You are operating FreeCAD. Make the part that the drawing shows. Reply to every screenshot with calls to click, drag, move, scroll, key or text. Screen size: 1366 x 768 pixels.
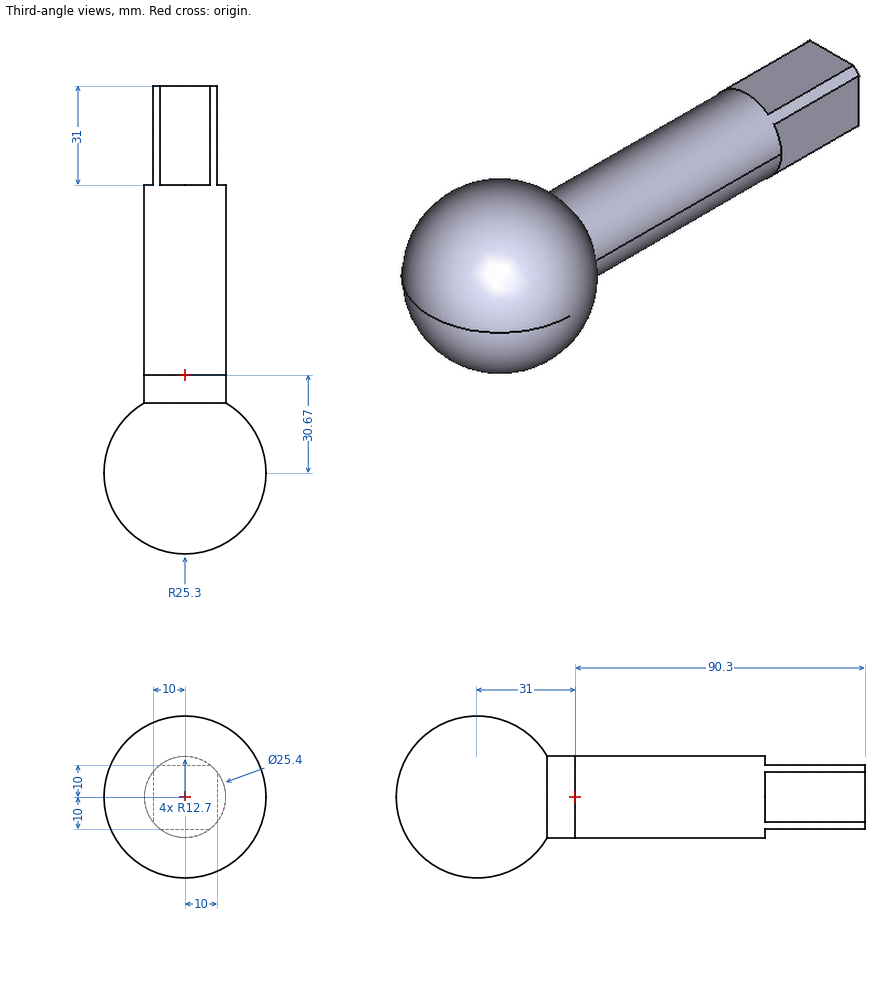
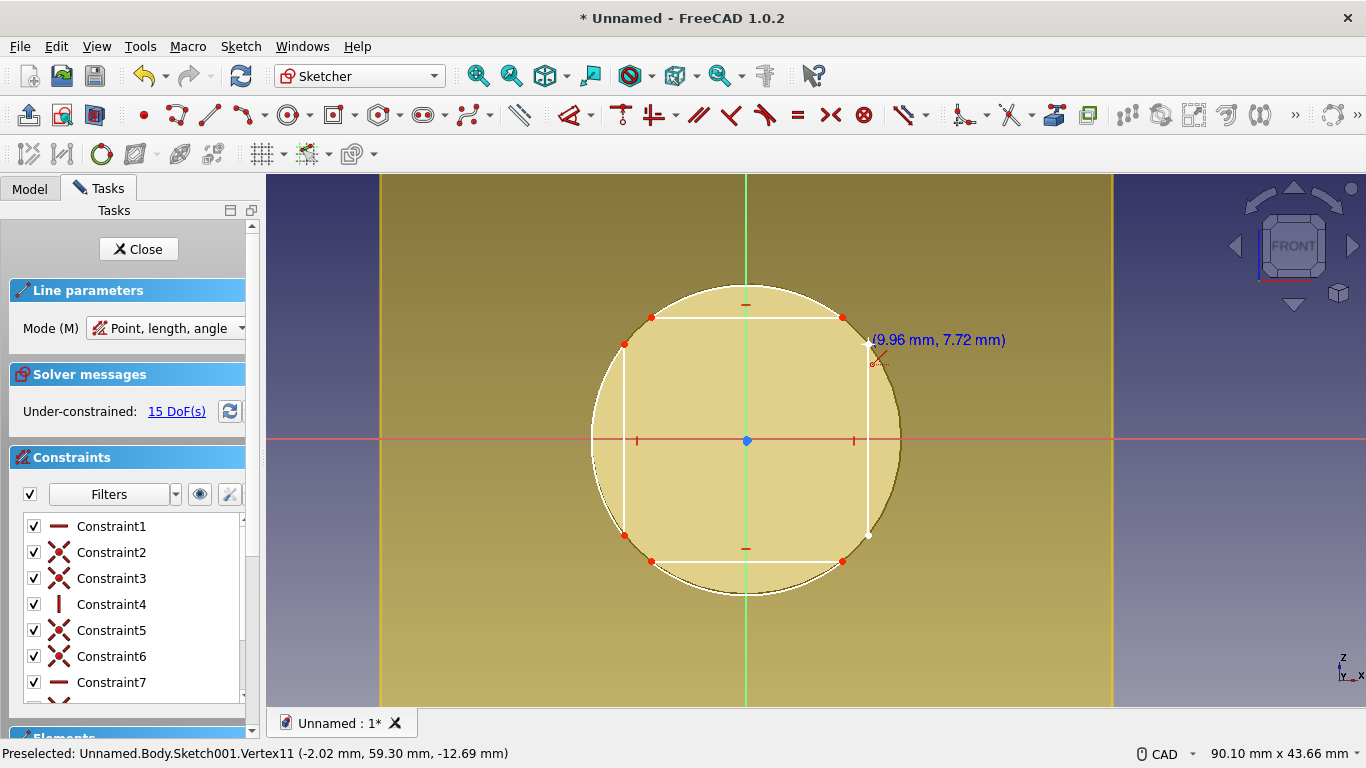
key(g)
key(3)
key(a)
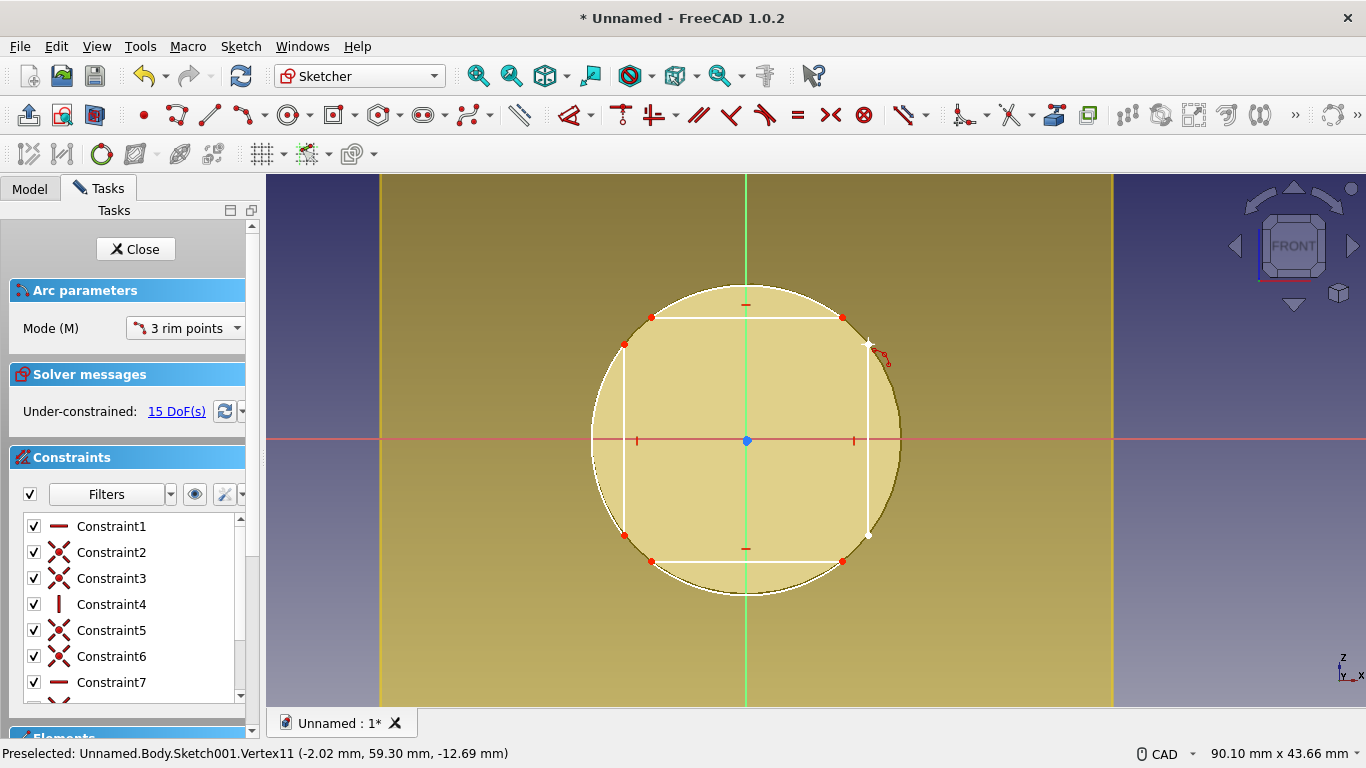
click(868, 345)
click(868, 536)
click(900, 460)
key(Escape)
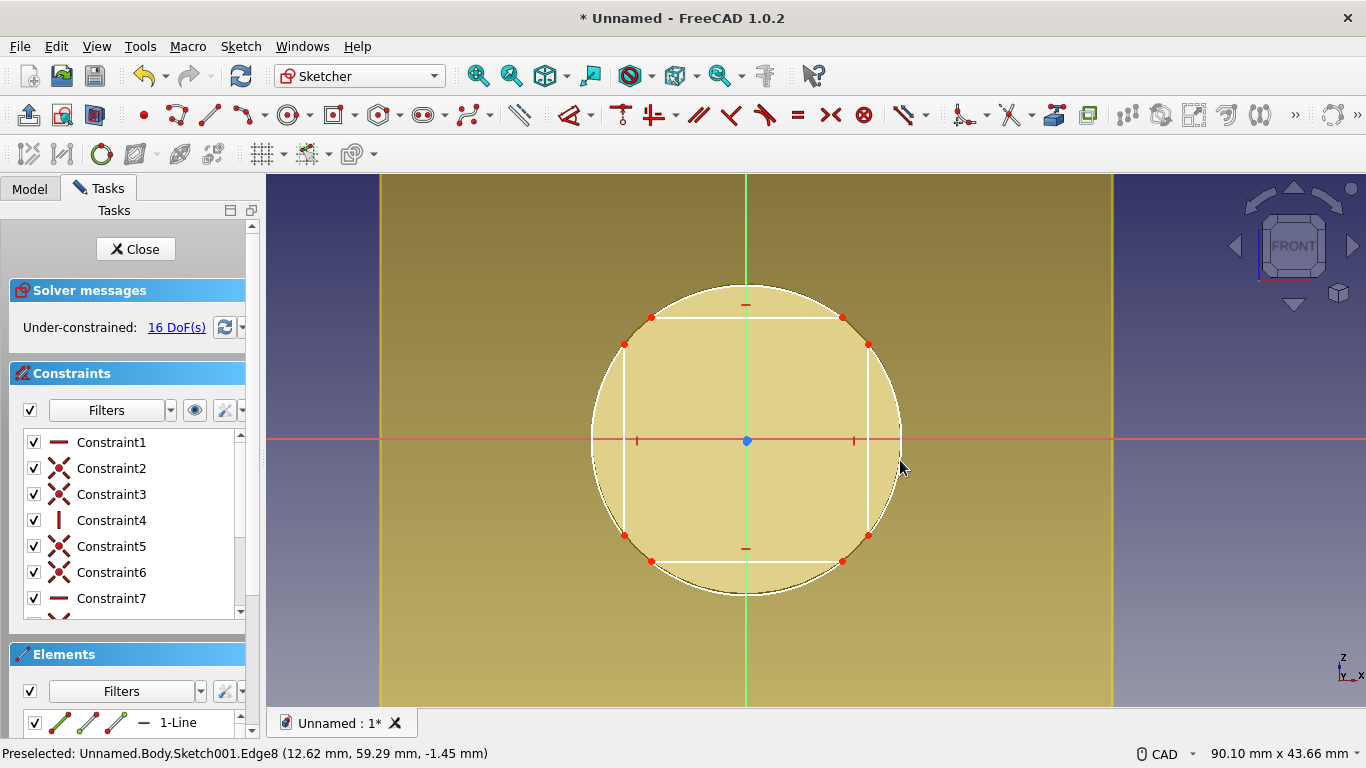
click(787, 291)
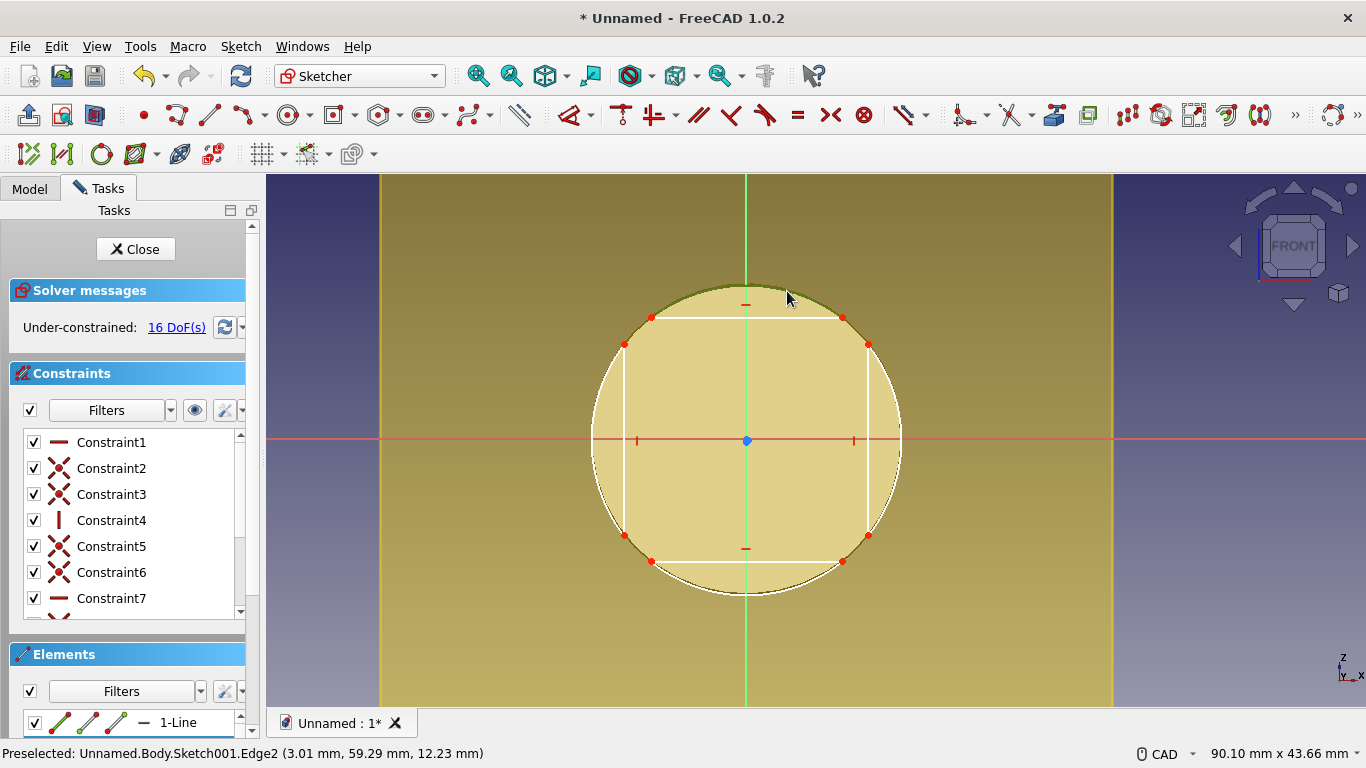
click(597, 400)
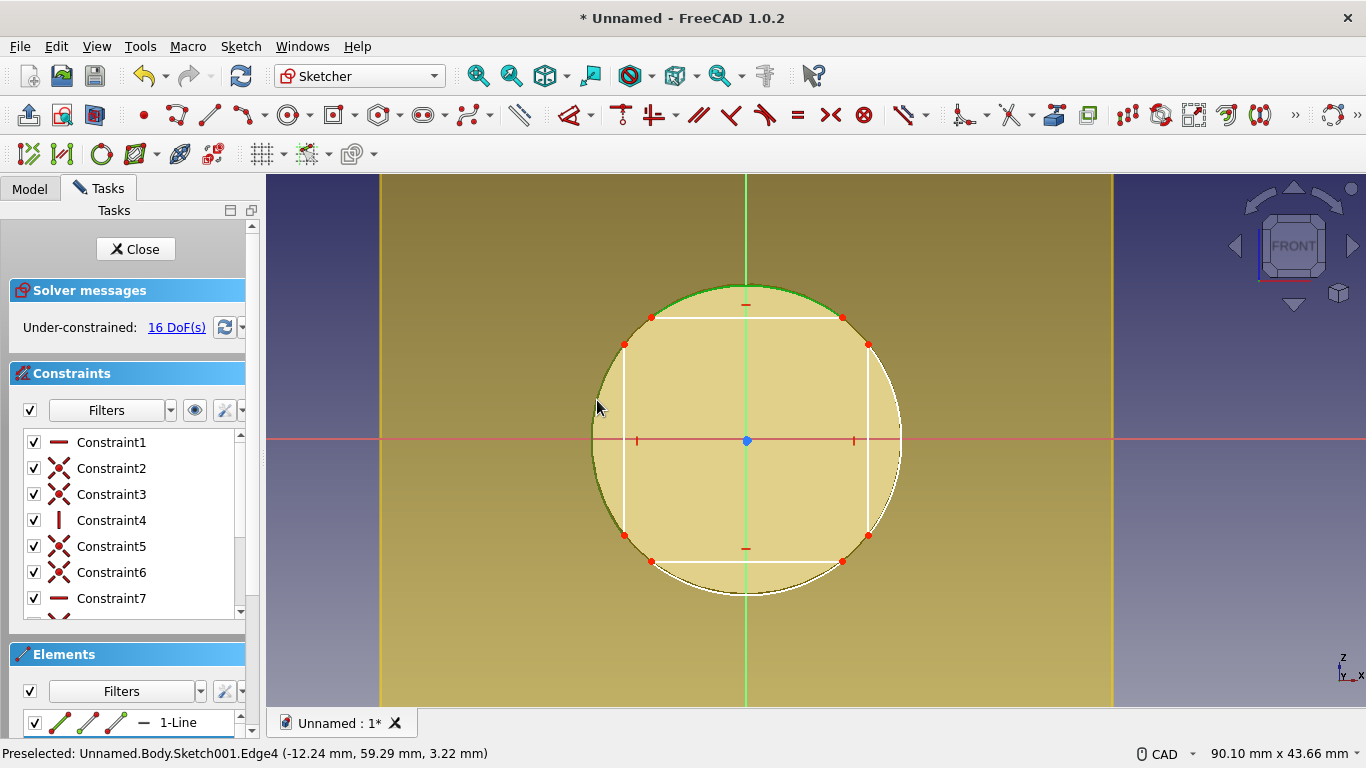
key(c)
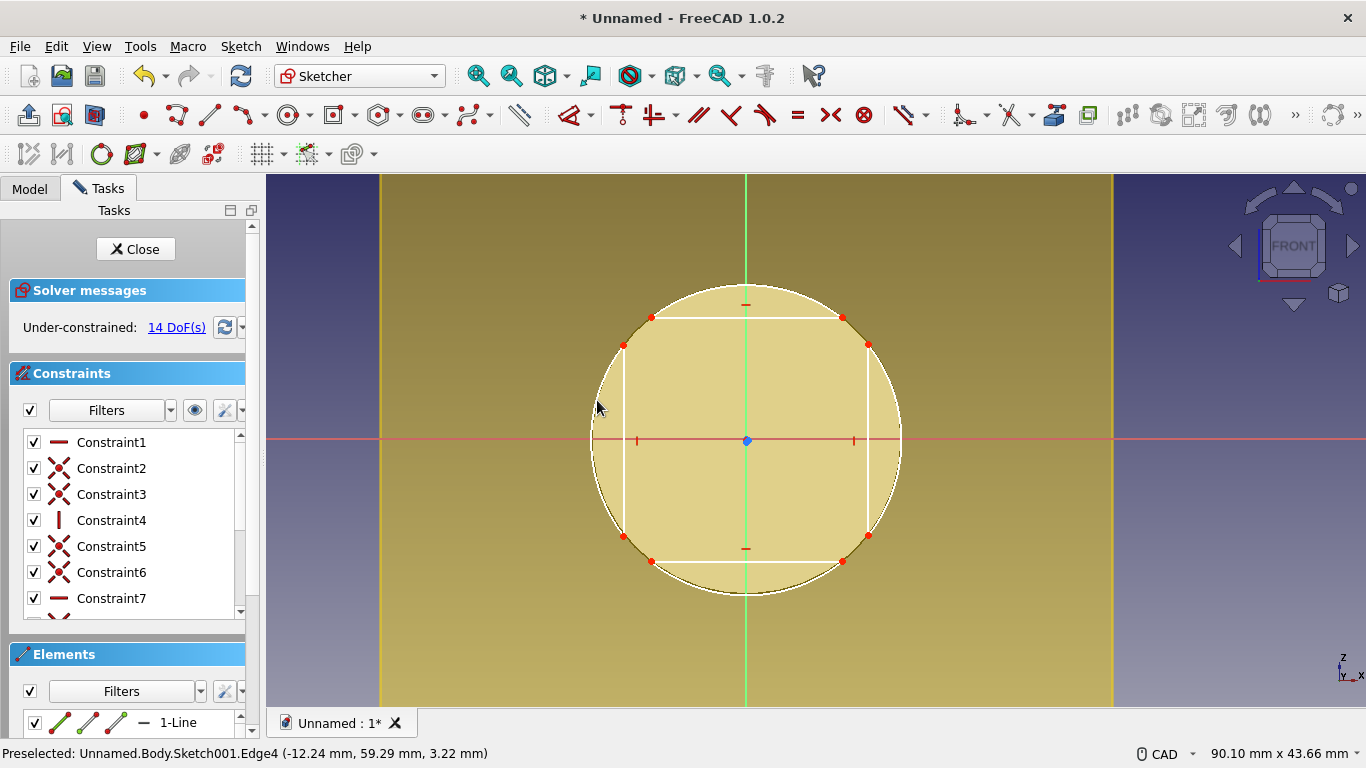
click(787, 291)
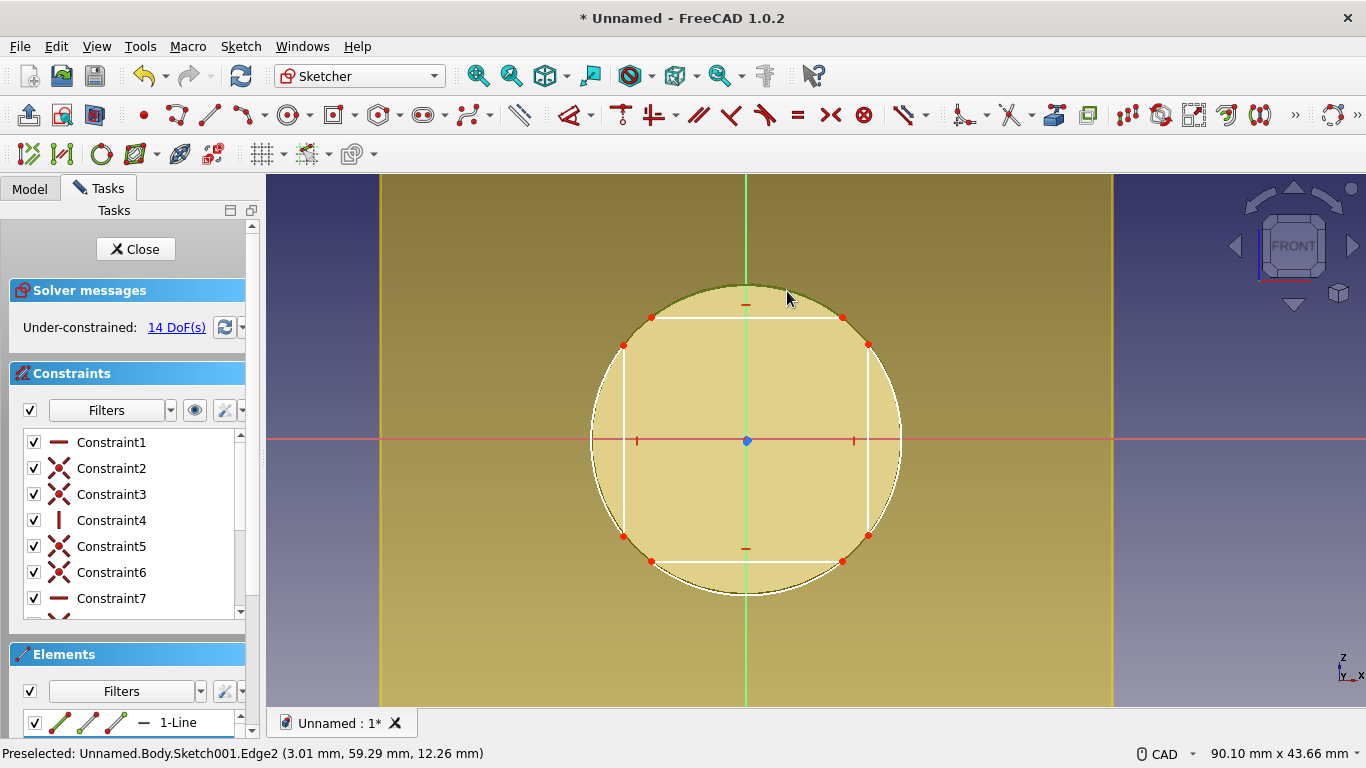
click(706, 590)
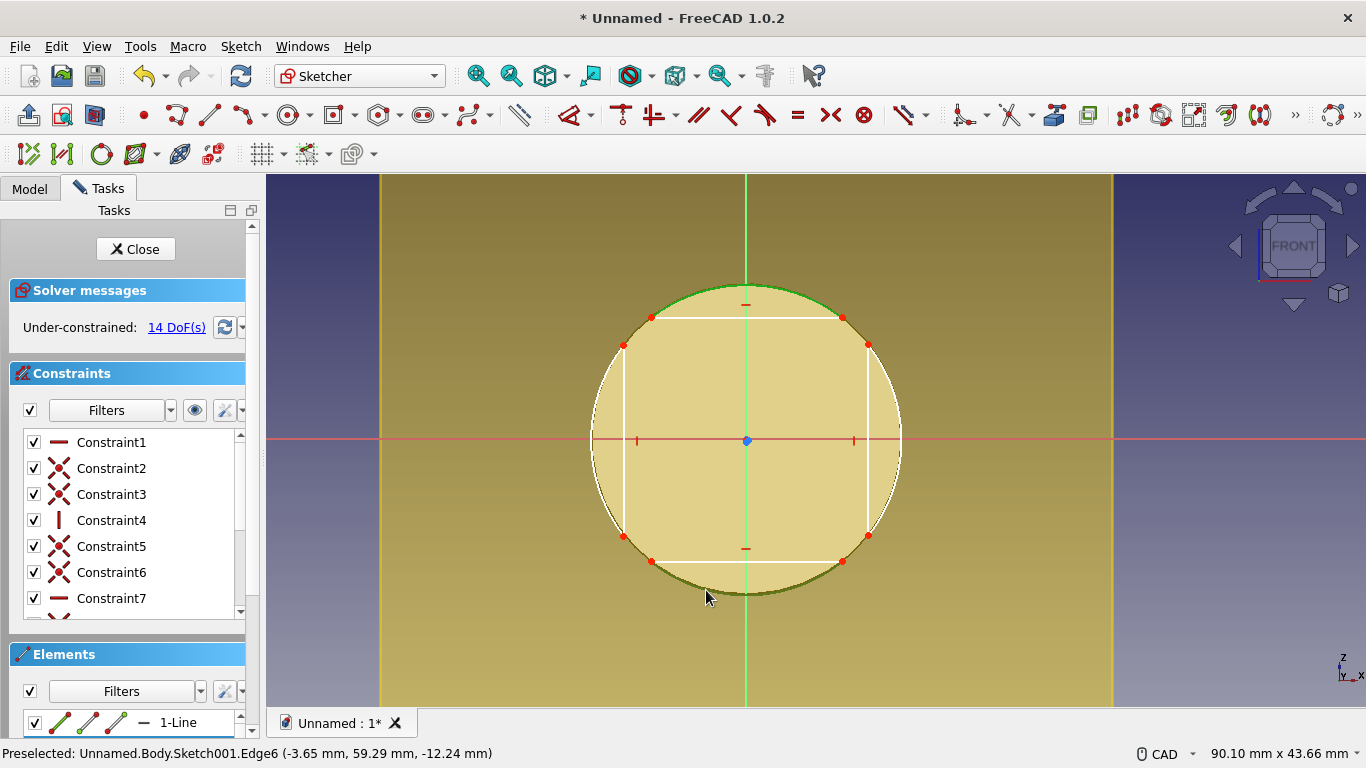
click(621, 116)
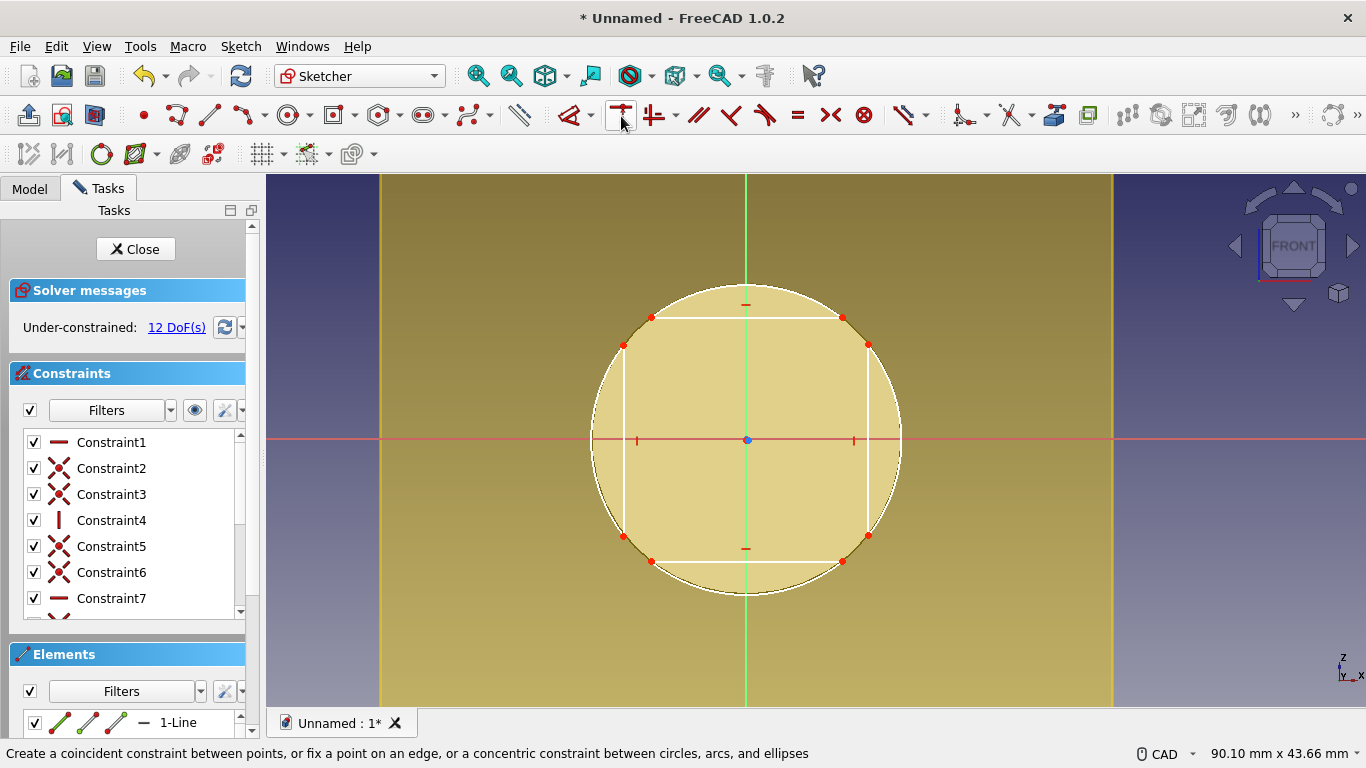
click(787, 291)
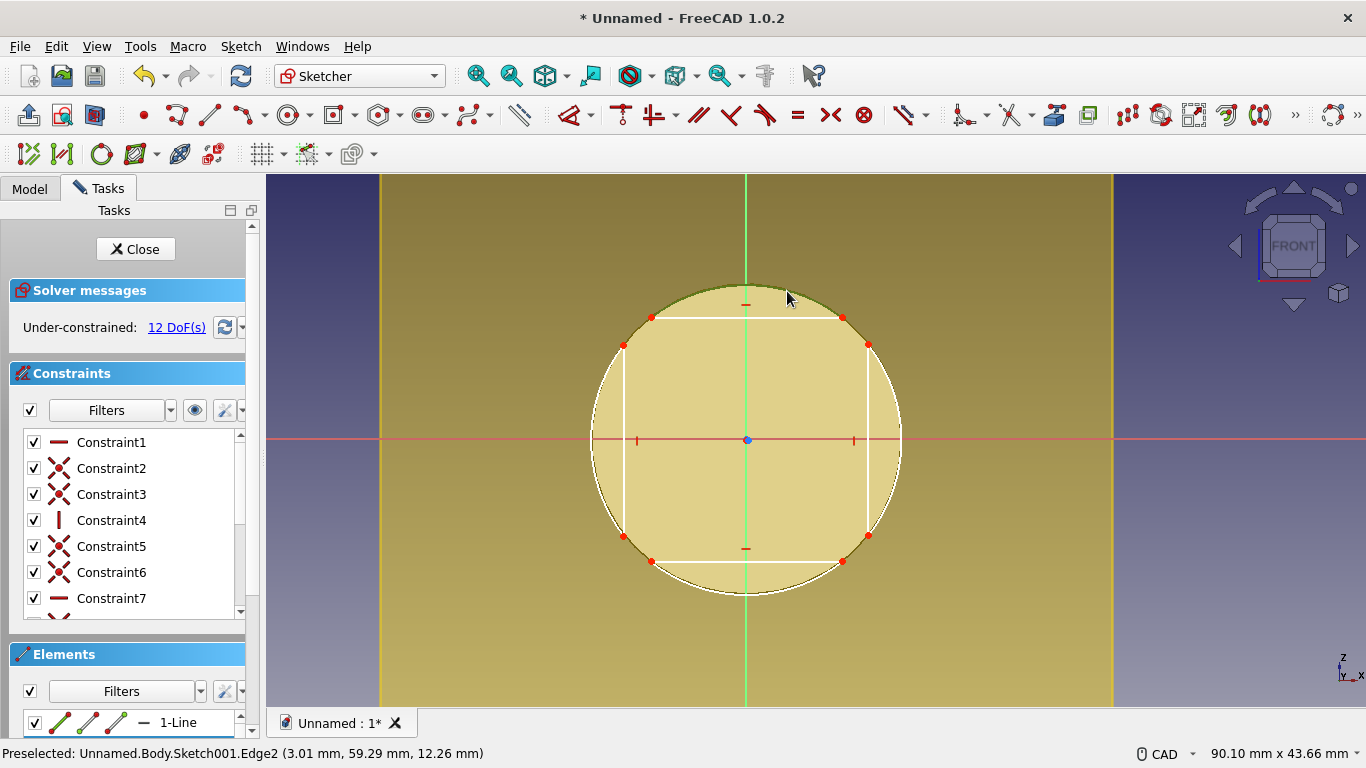
click(896, 481)